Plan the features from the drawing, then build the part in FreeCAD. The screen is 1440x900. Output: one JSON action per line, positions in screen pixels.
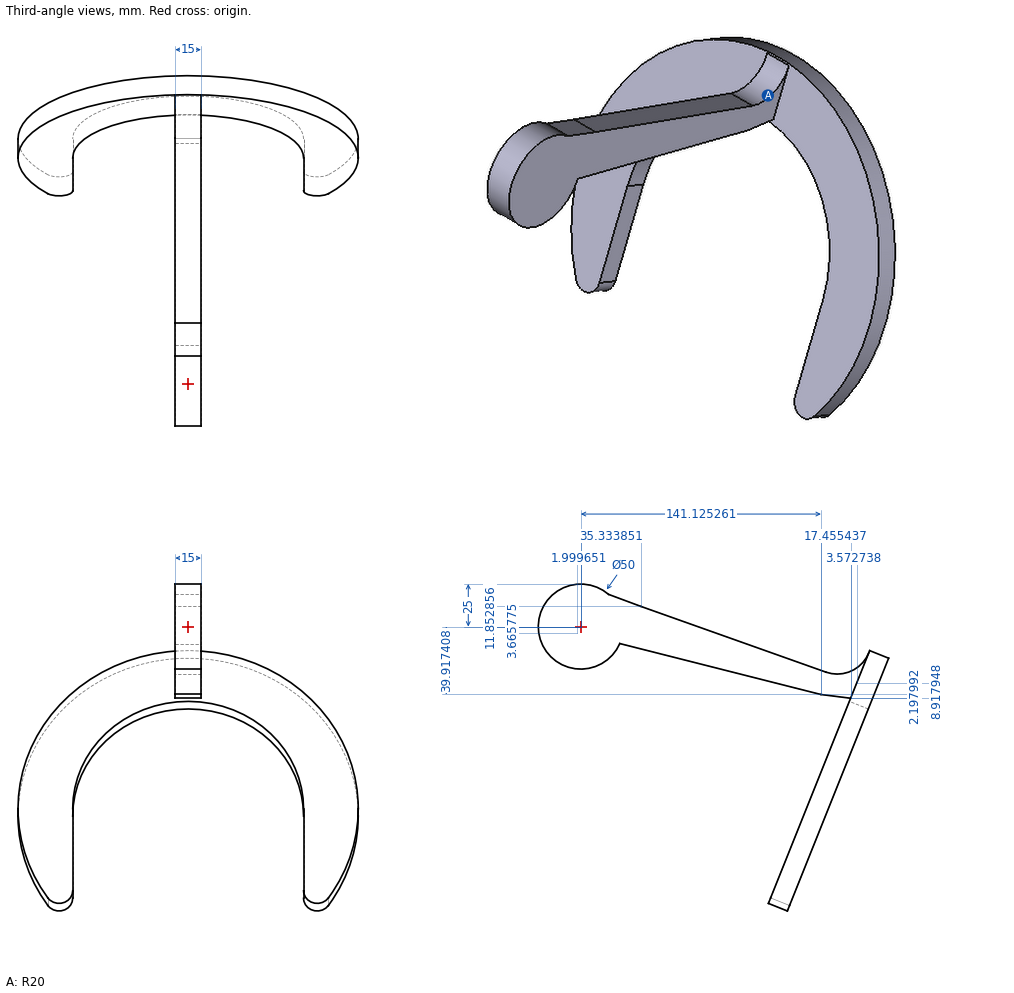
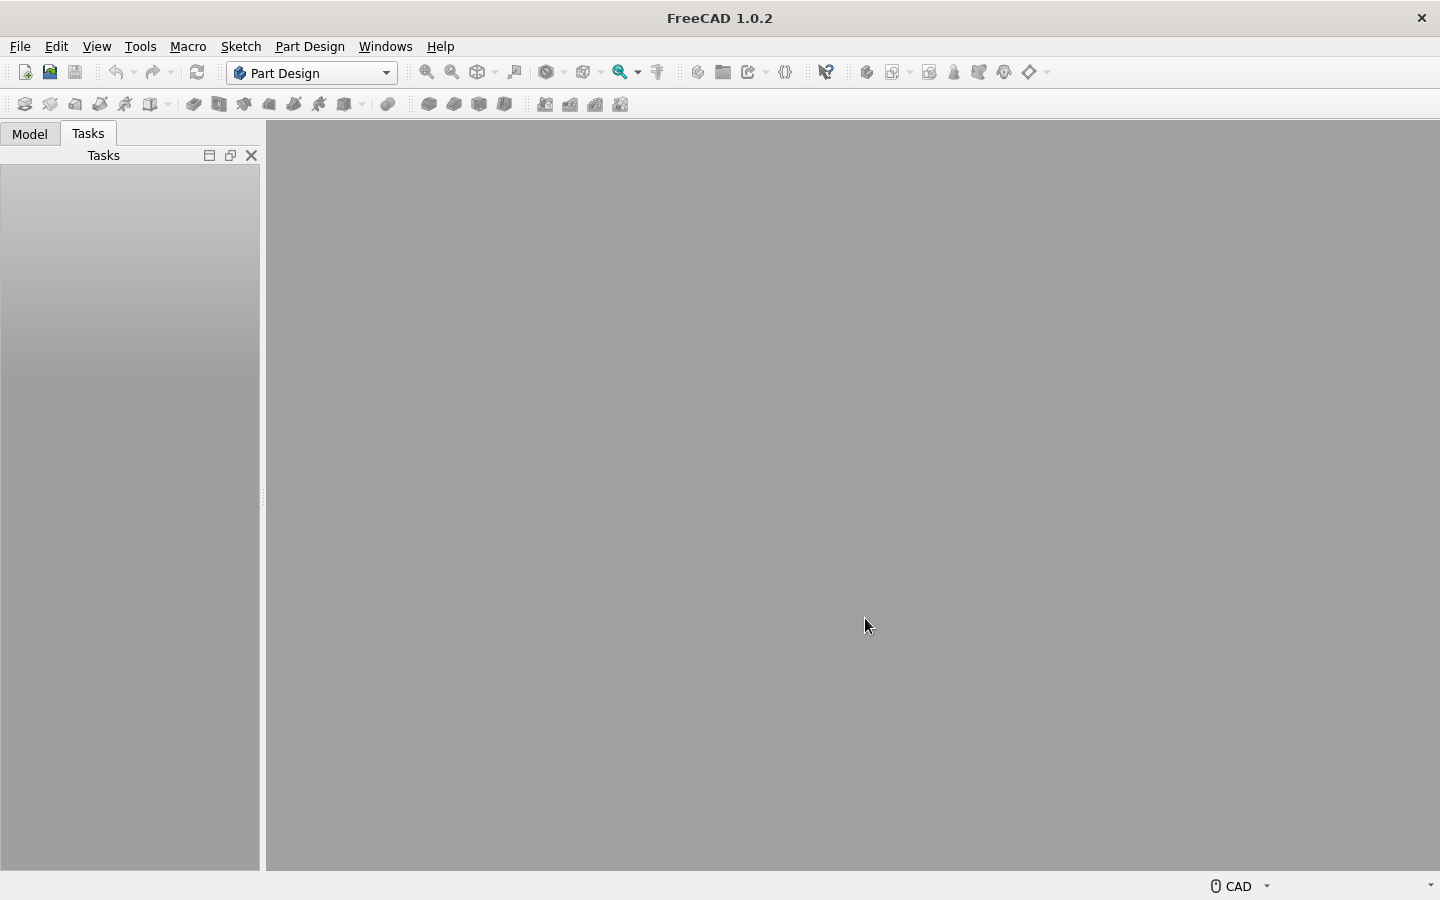
{"action": "key", "text": "ctrl+n"}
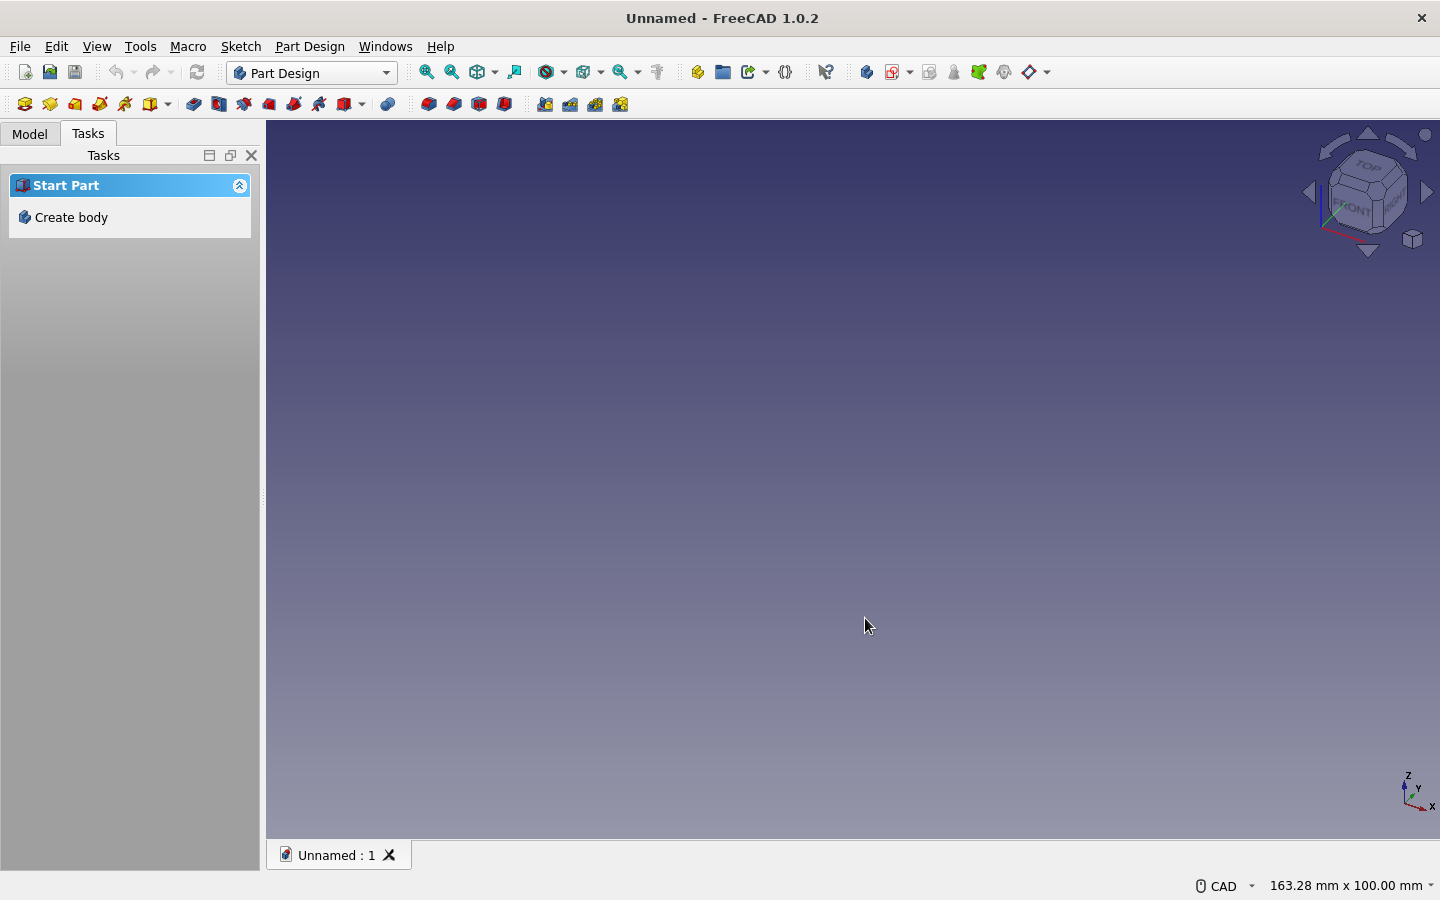
{"action": "left_click", "coordinate": [892, 72]}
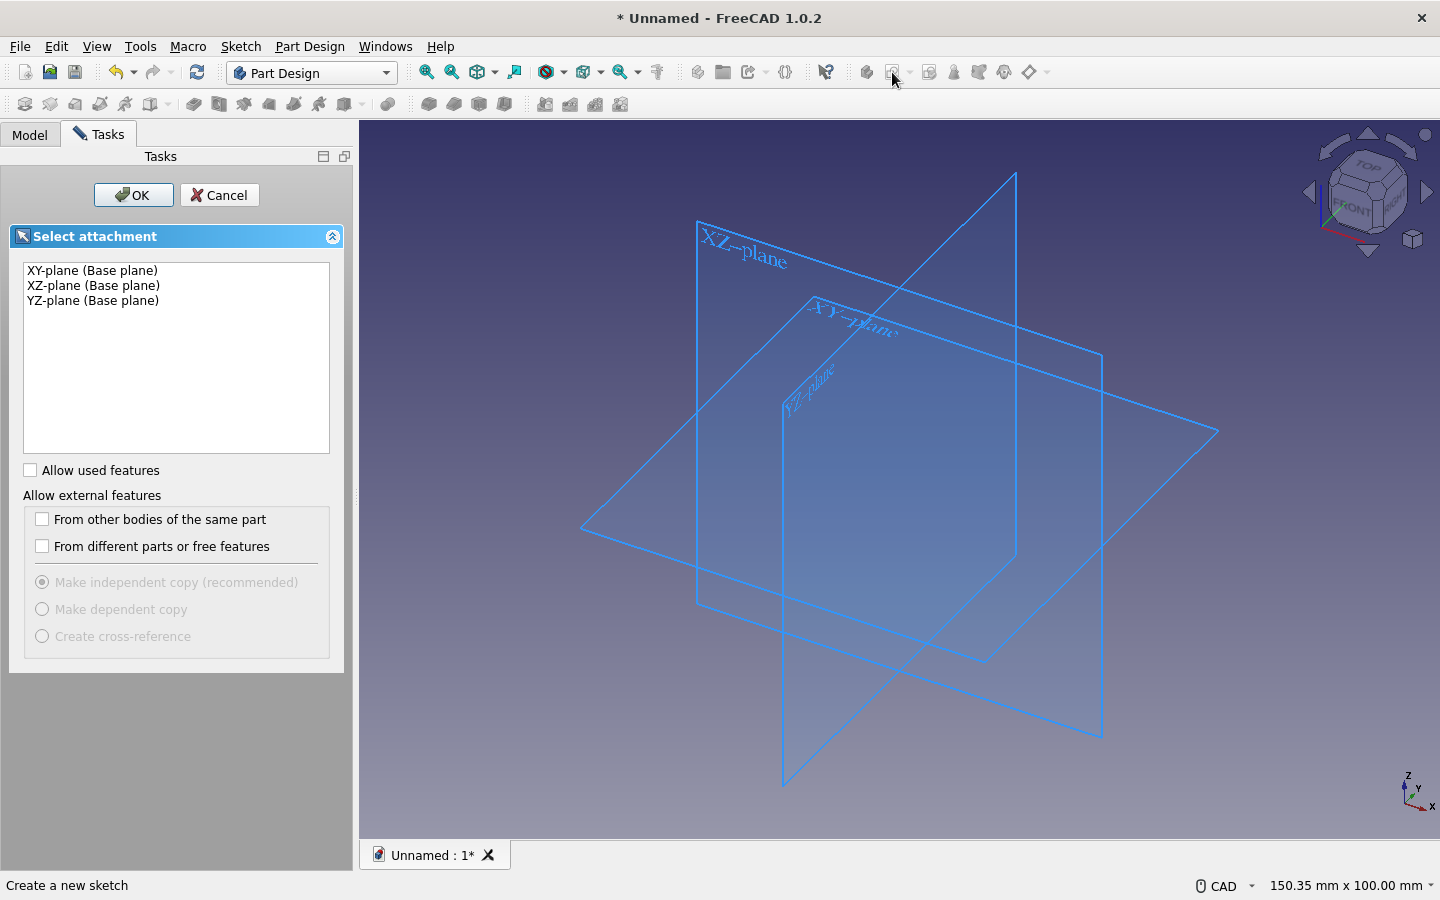
{"action": "left_click", "coordinate": [84, 300]}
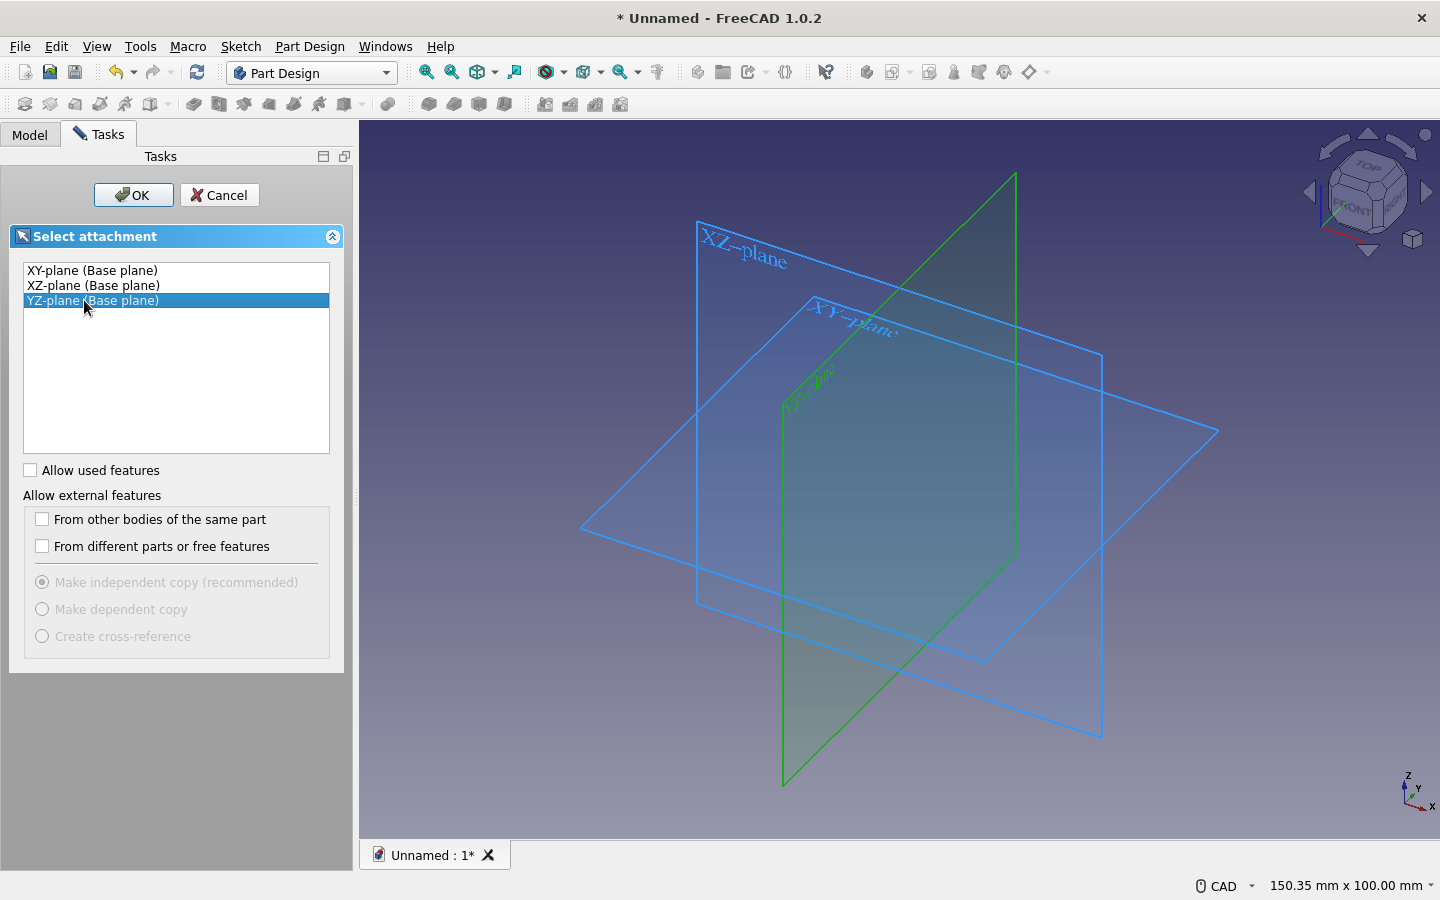
{"action": "left_click", "coordinate": [134, 195]}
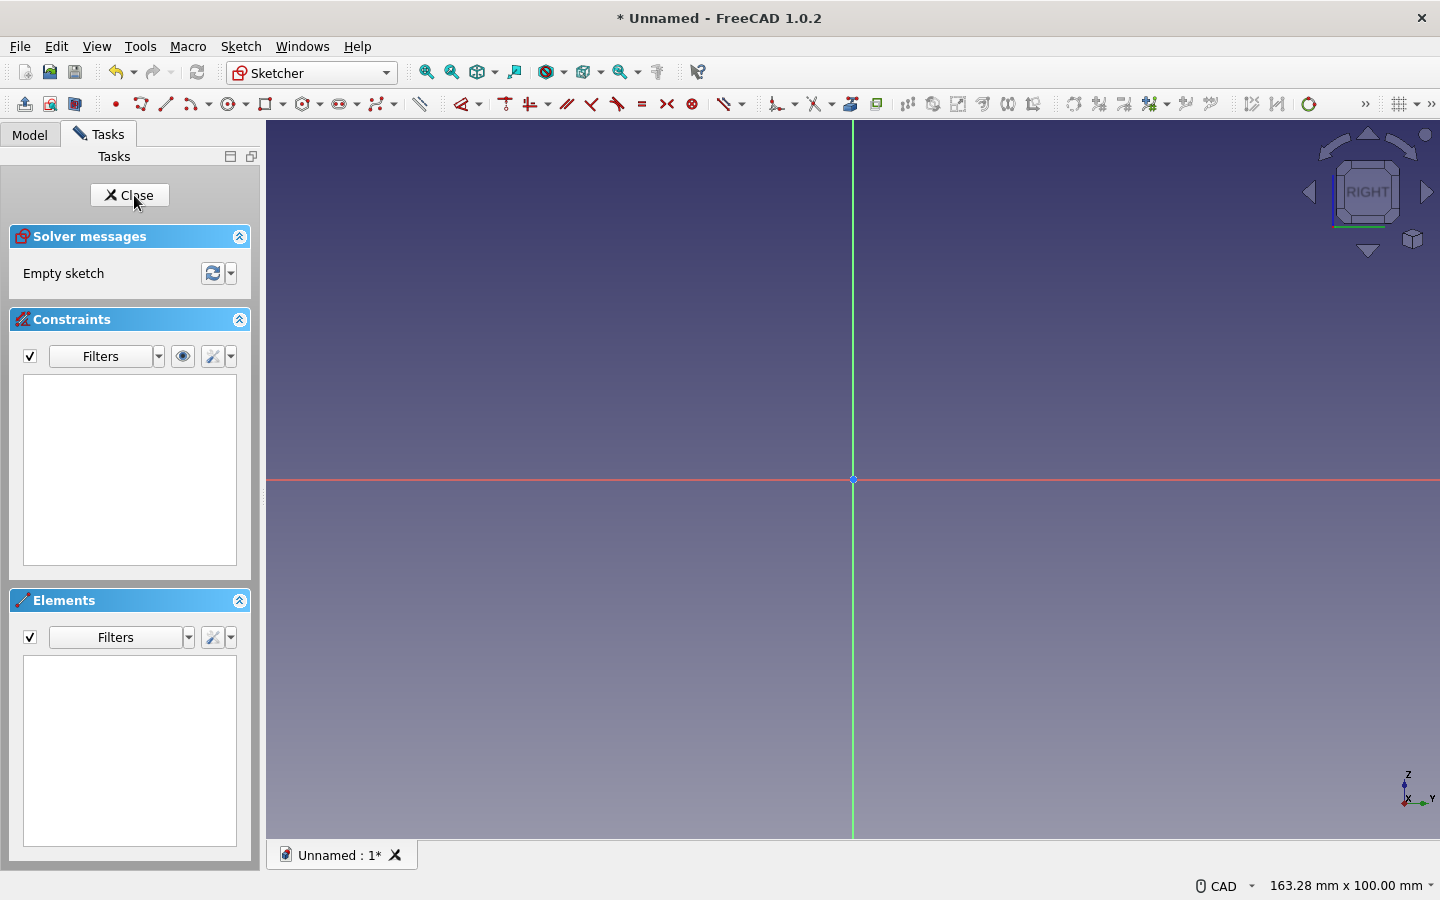
{"action": "left_click", "coordinate": [228, 104]}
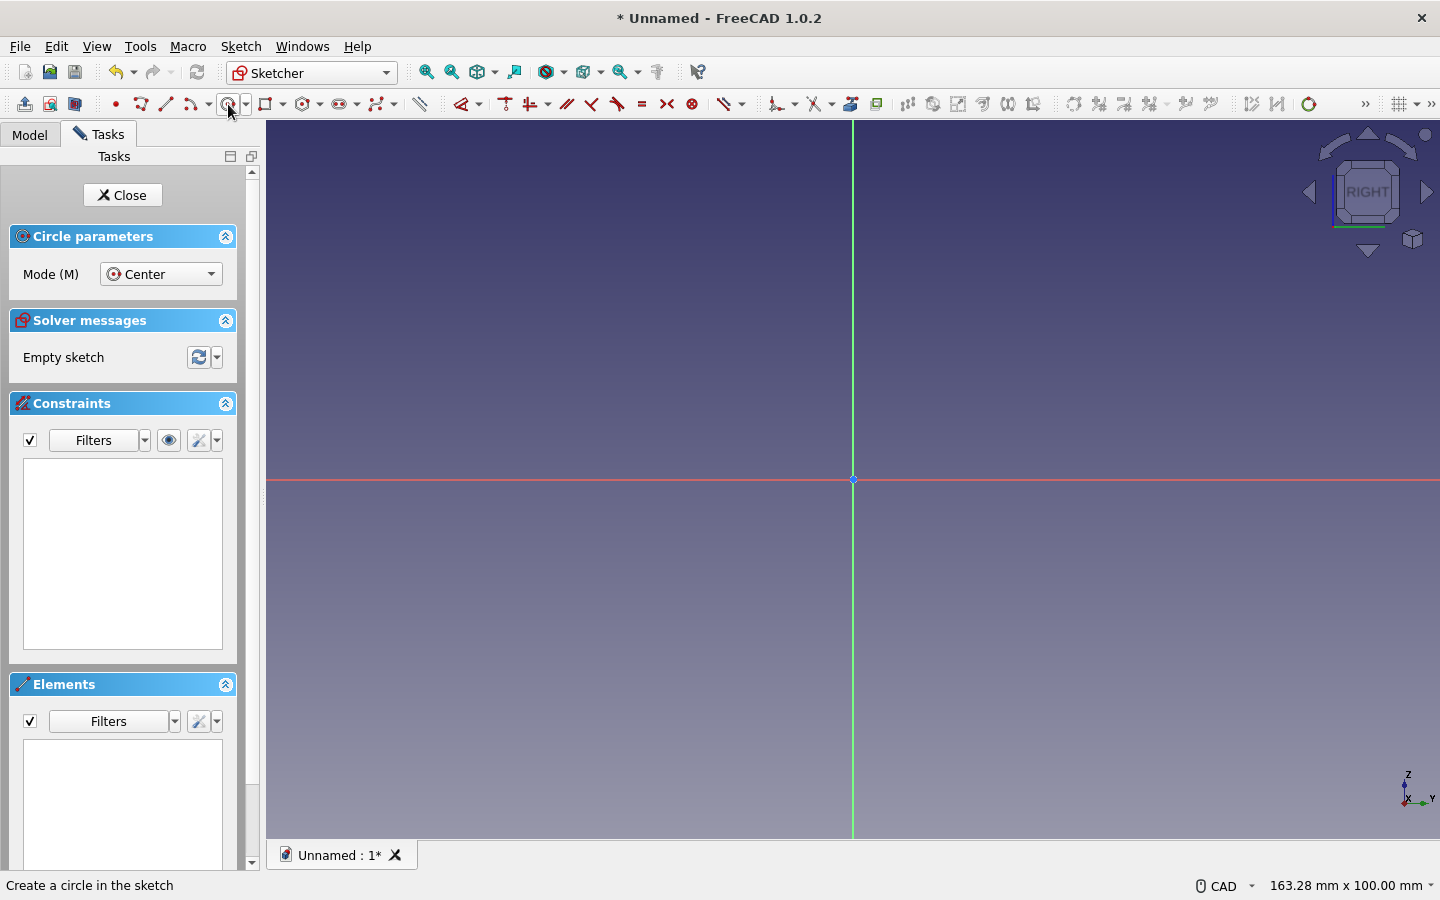
{"action": "left_click", "coordinate": [853, 480]}
{"action": "left_click", "coordinate": [980, 352]}
{"action": "key", "text": "Escape"}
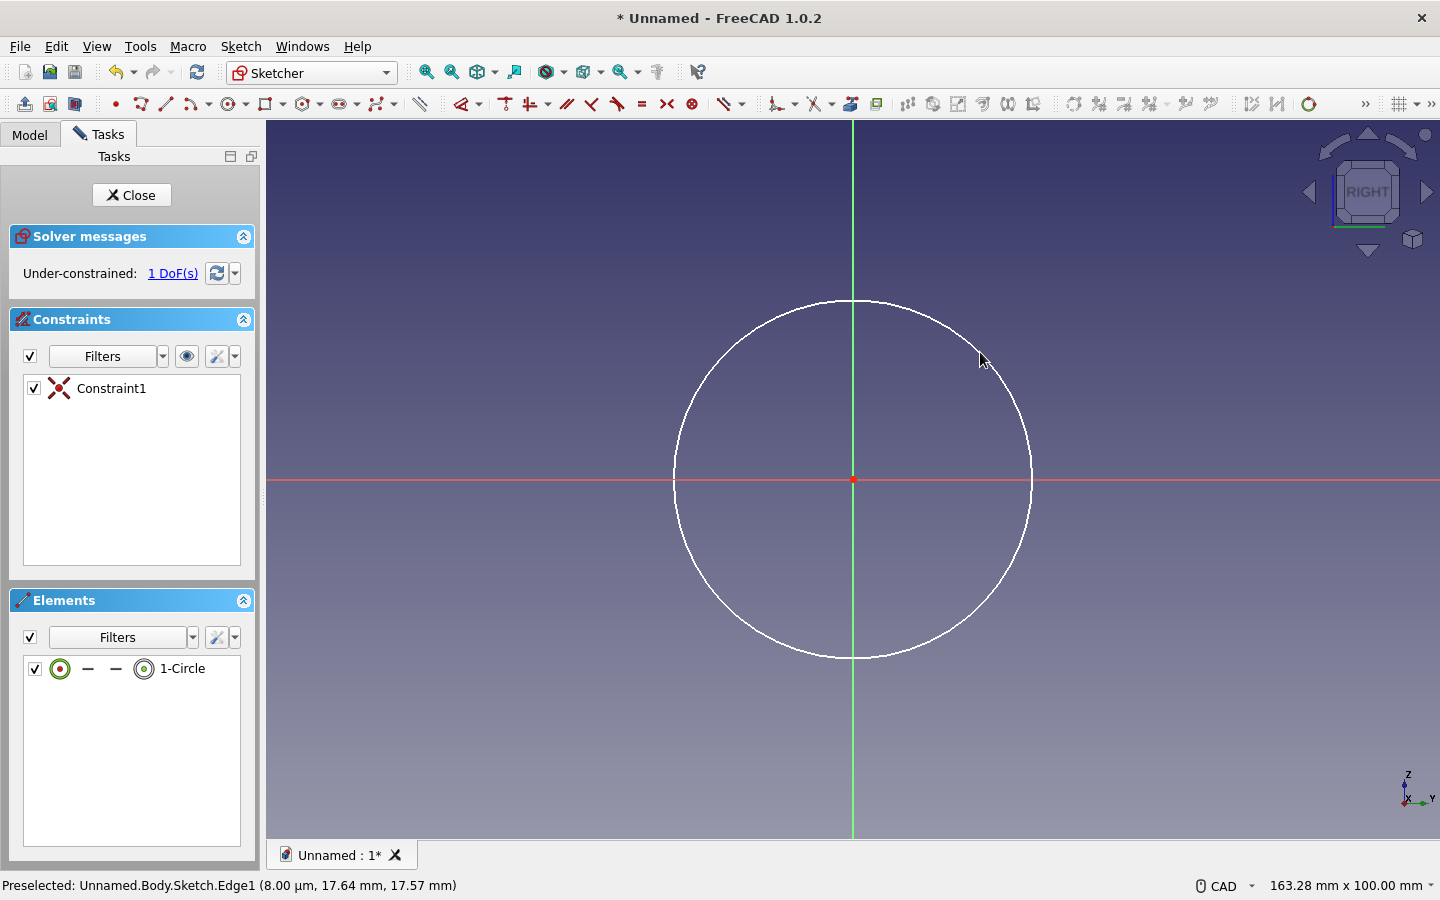
{"action": "key", "text": "d"}